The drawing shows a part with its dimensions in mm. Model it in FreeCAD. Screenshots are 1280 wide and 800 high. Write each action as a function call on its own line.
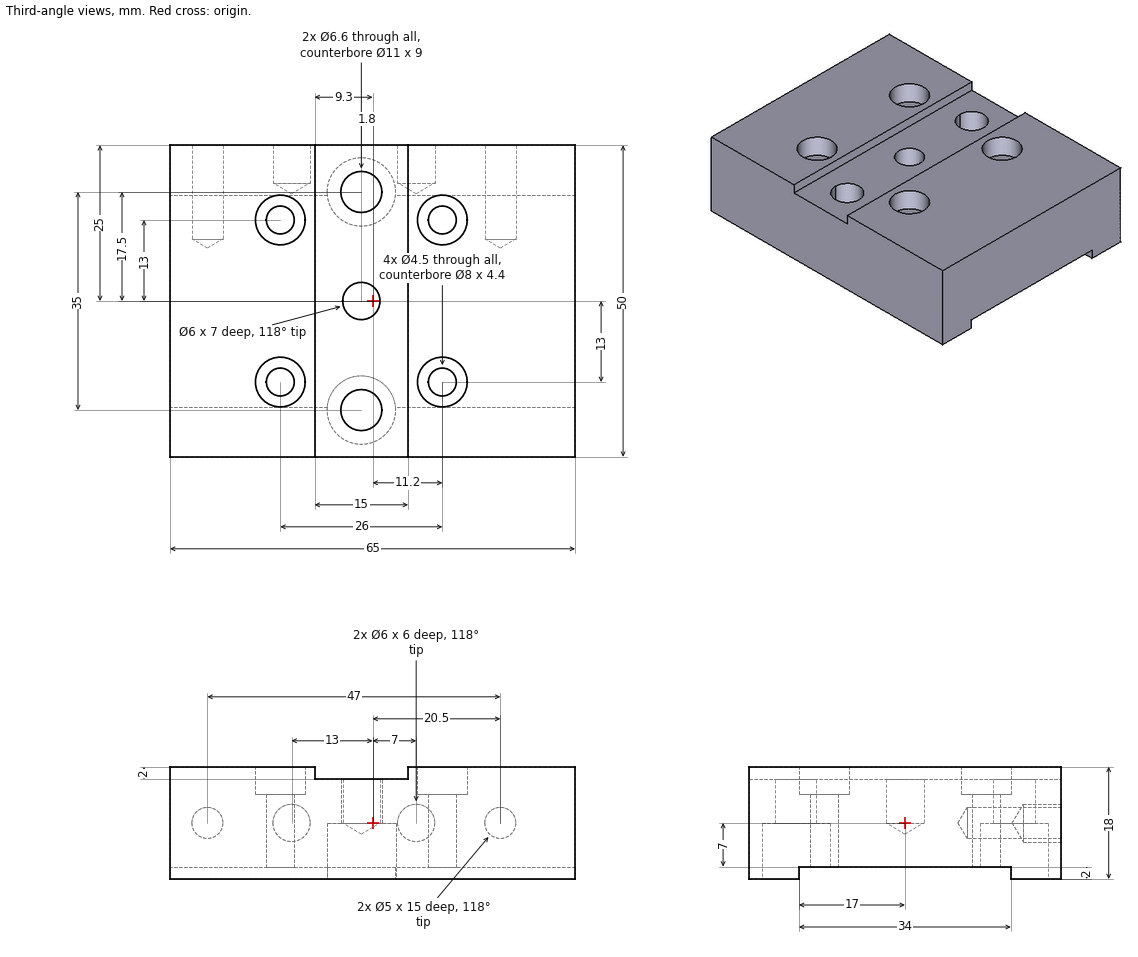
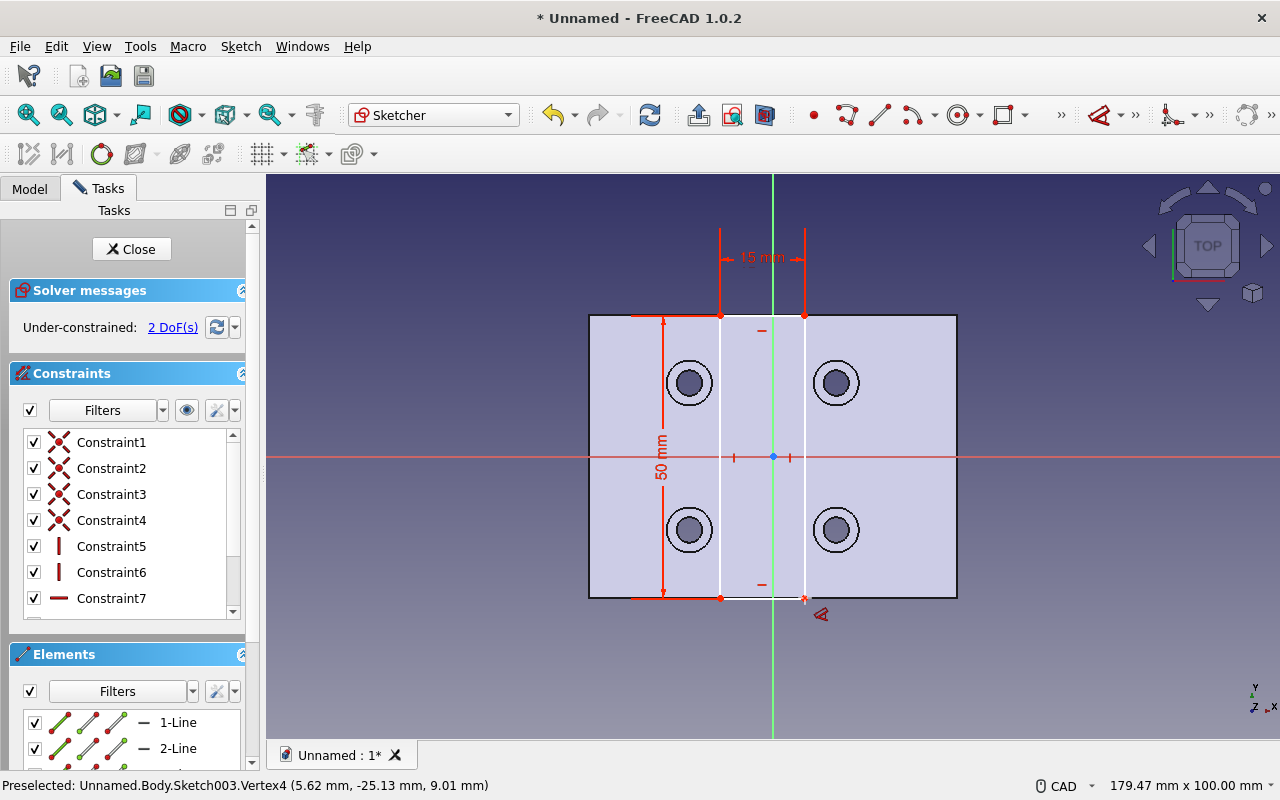
click(720, 316)
click(686, 386)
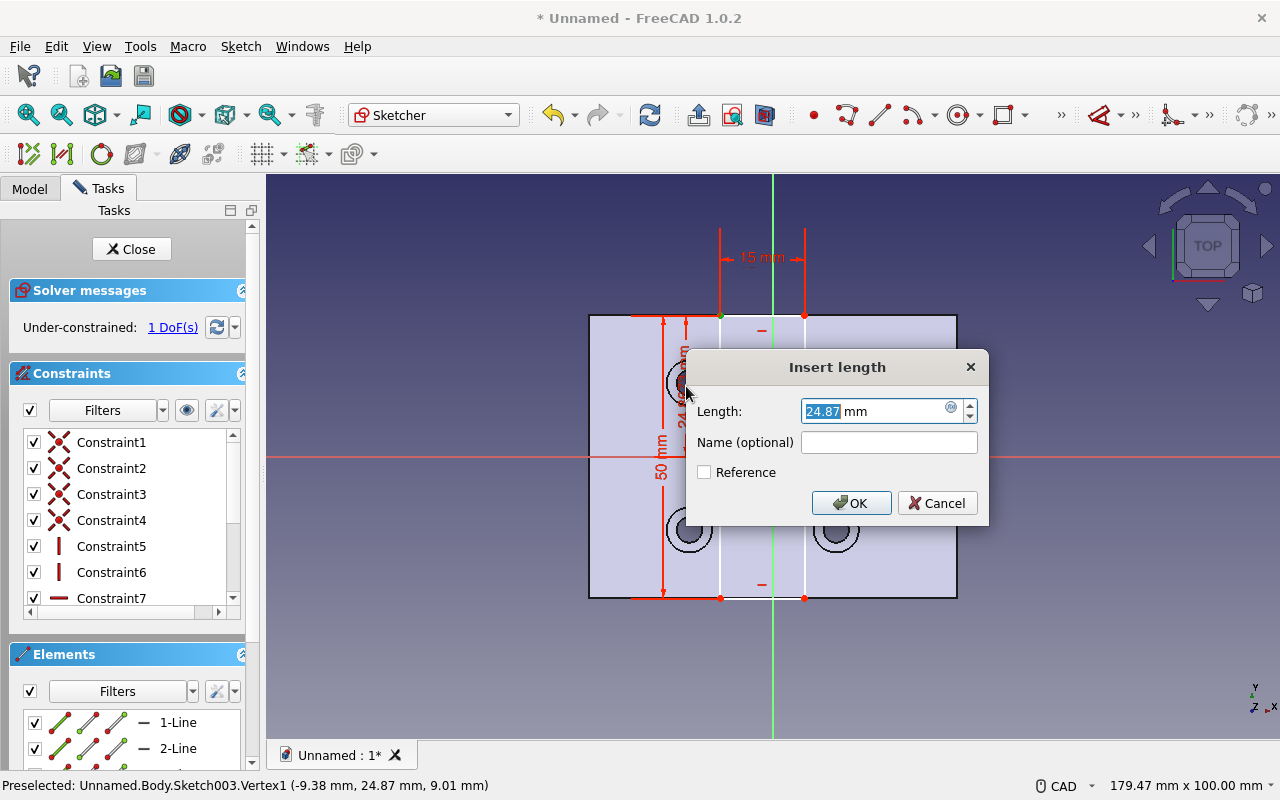
text(25)
key(Return)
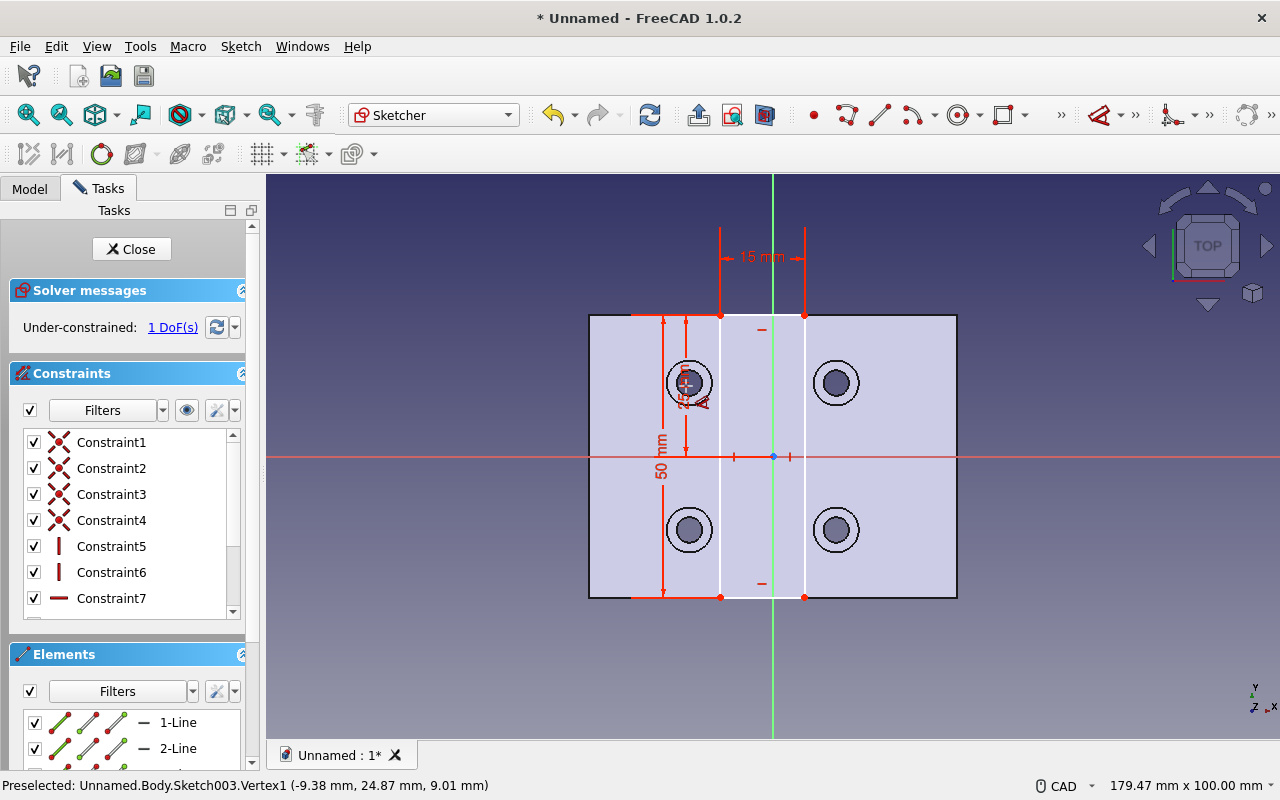
click(720, 315)
click(746, 281)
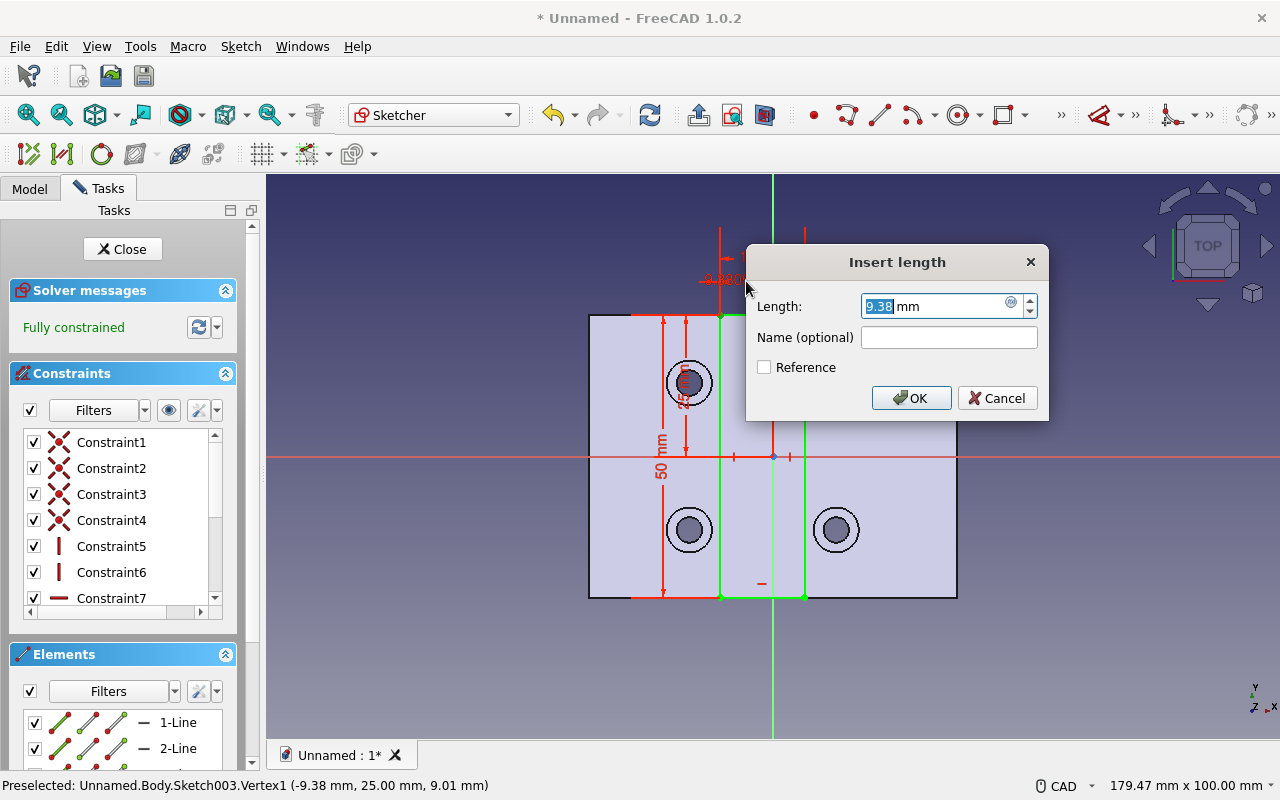
text(9.3)
key(Return)
key(Escape)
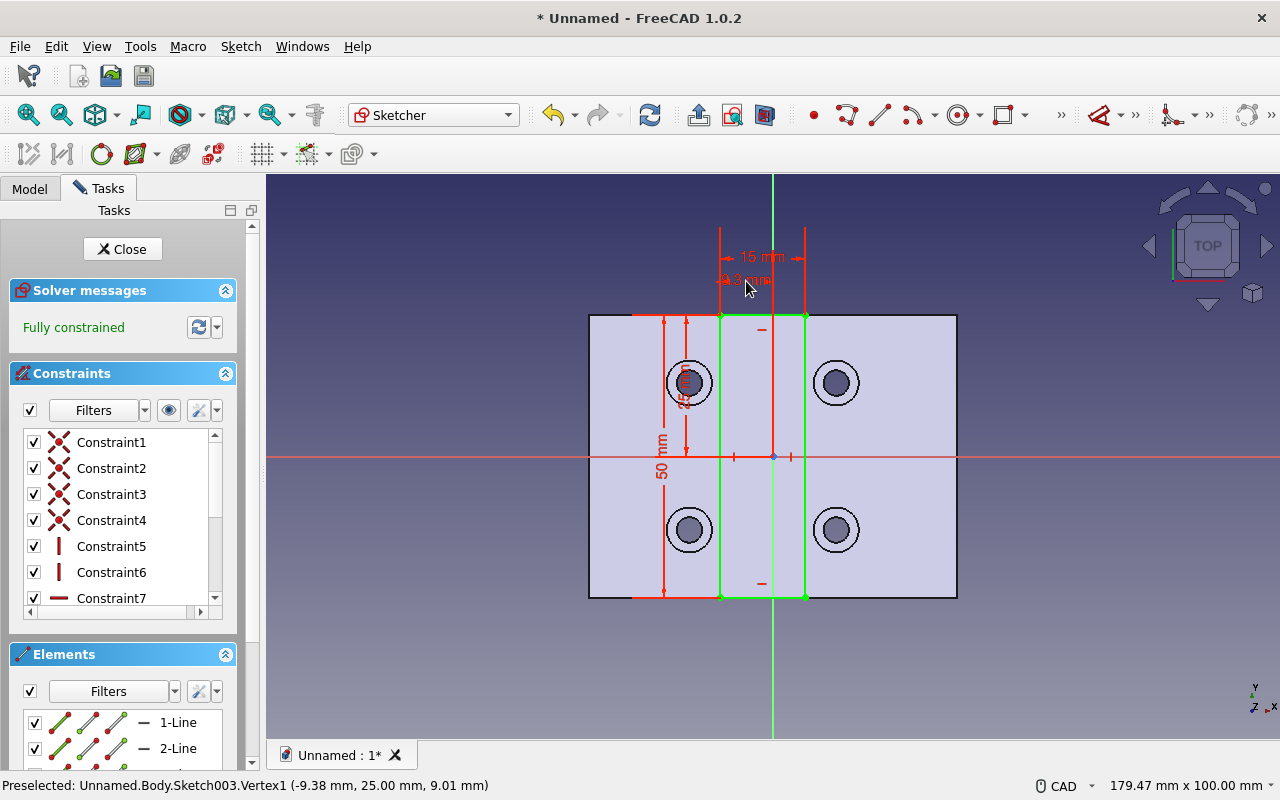
click(123, 249)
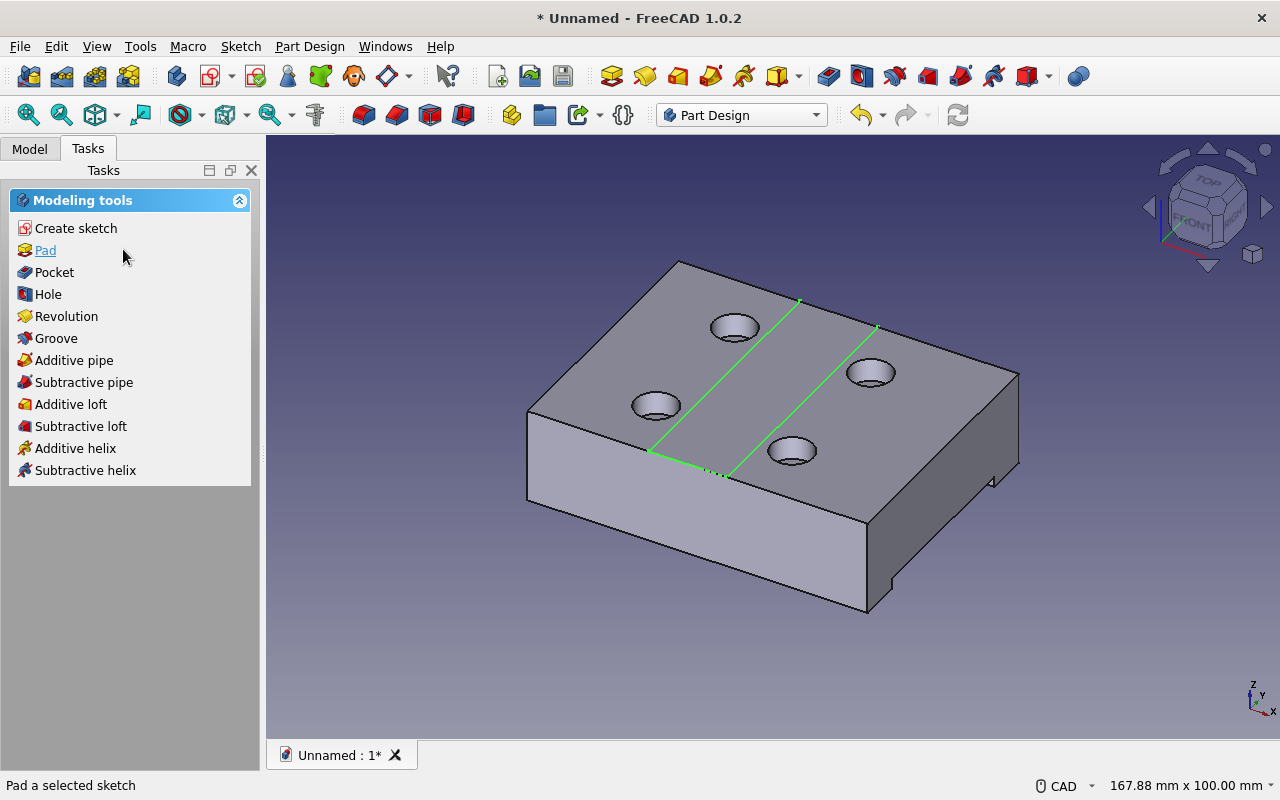
click(829, 76)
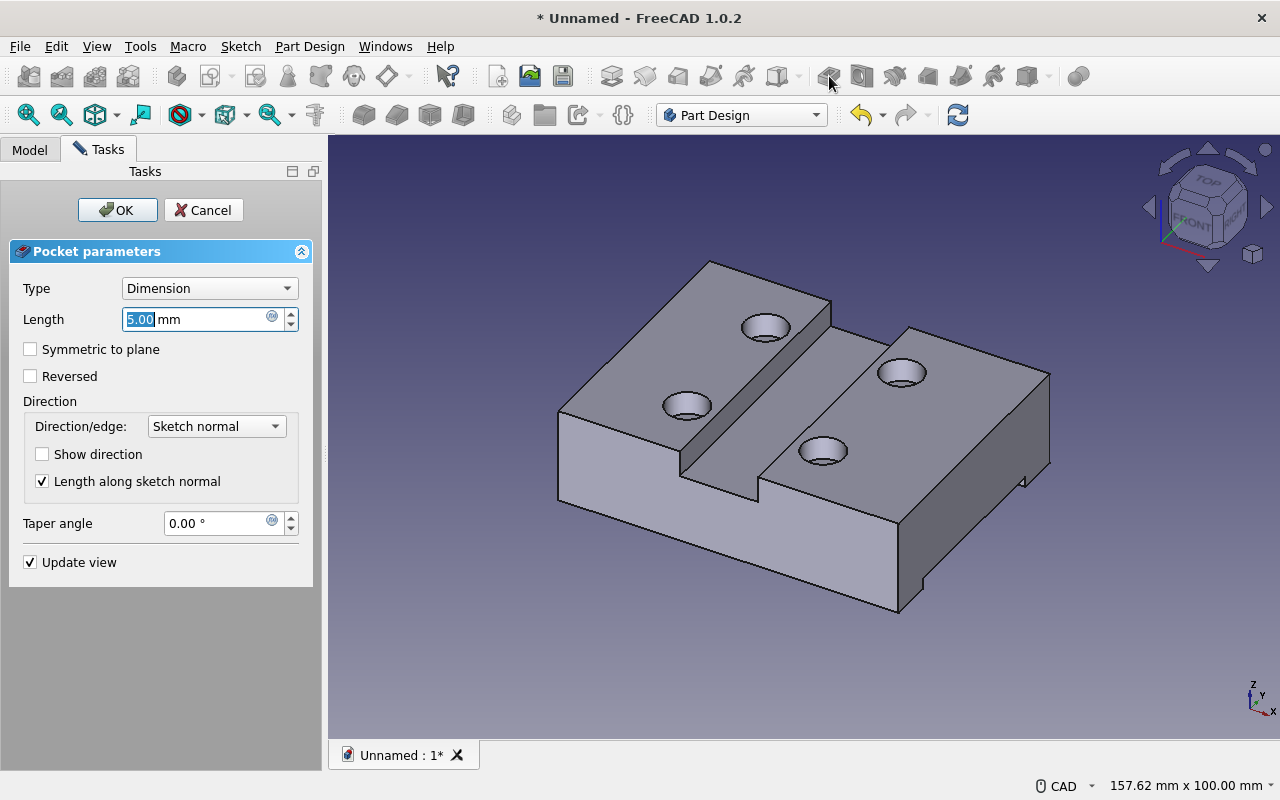
text(2)
key(Tab)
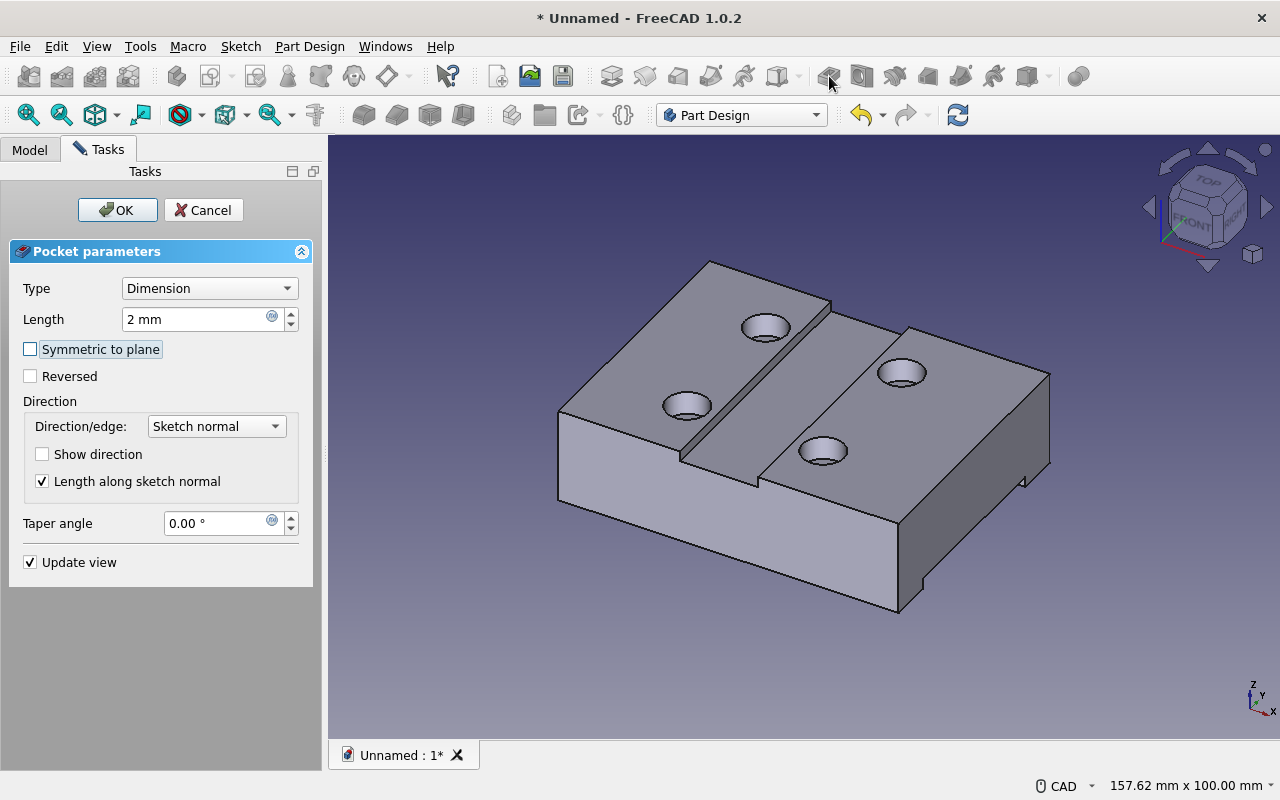
click(118, 210)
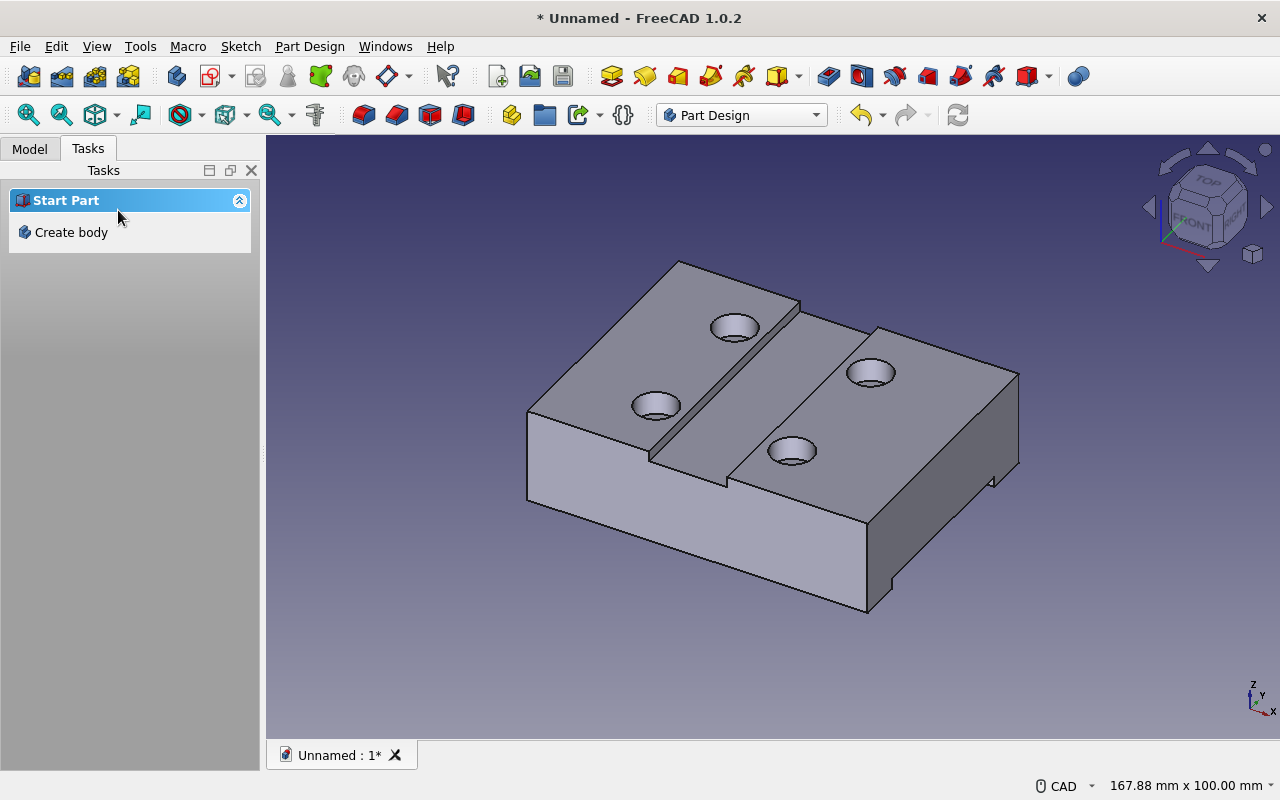
click(807, 355)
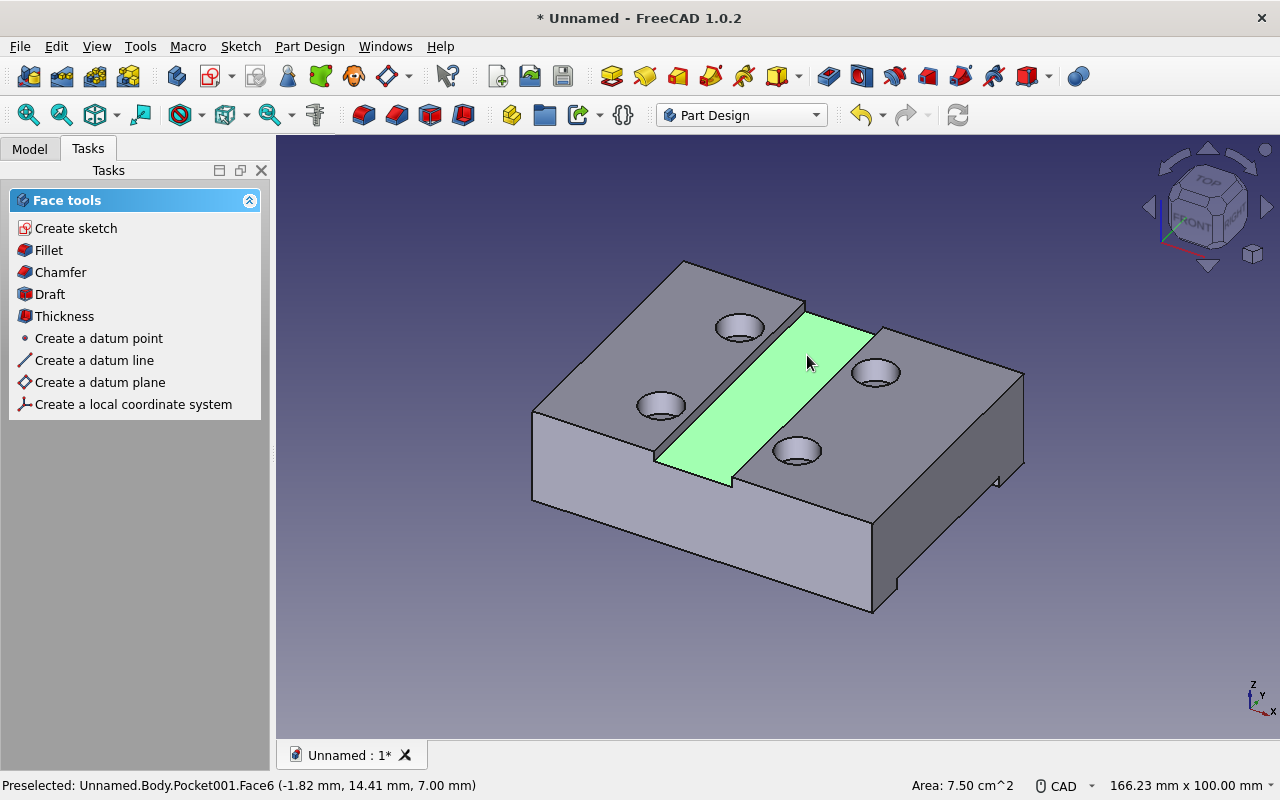
click(210, 76)